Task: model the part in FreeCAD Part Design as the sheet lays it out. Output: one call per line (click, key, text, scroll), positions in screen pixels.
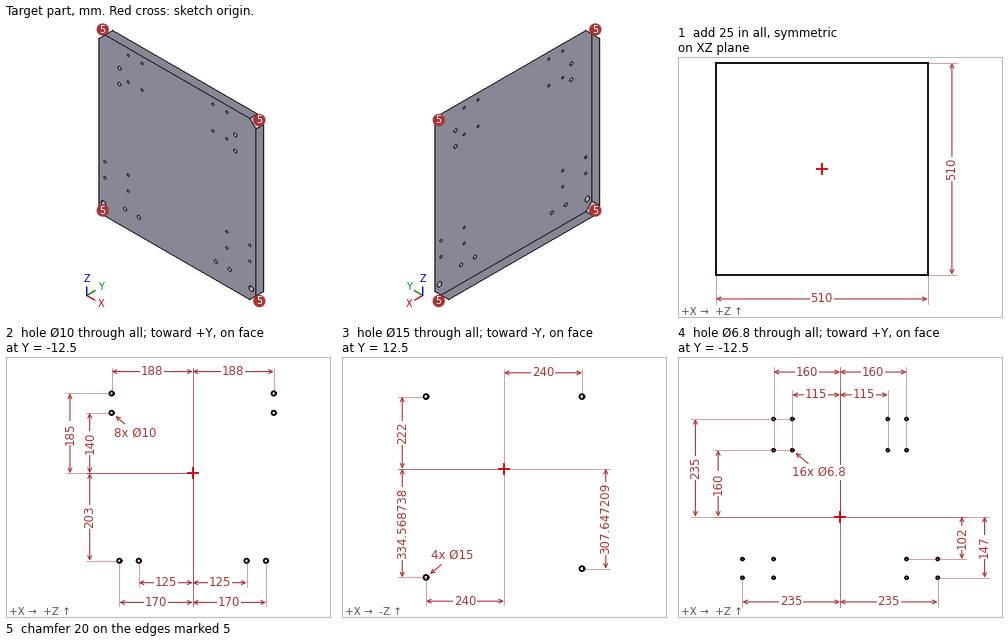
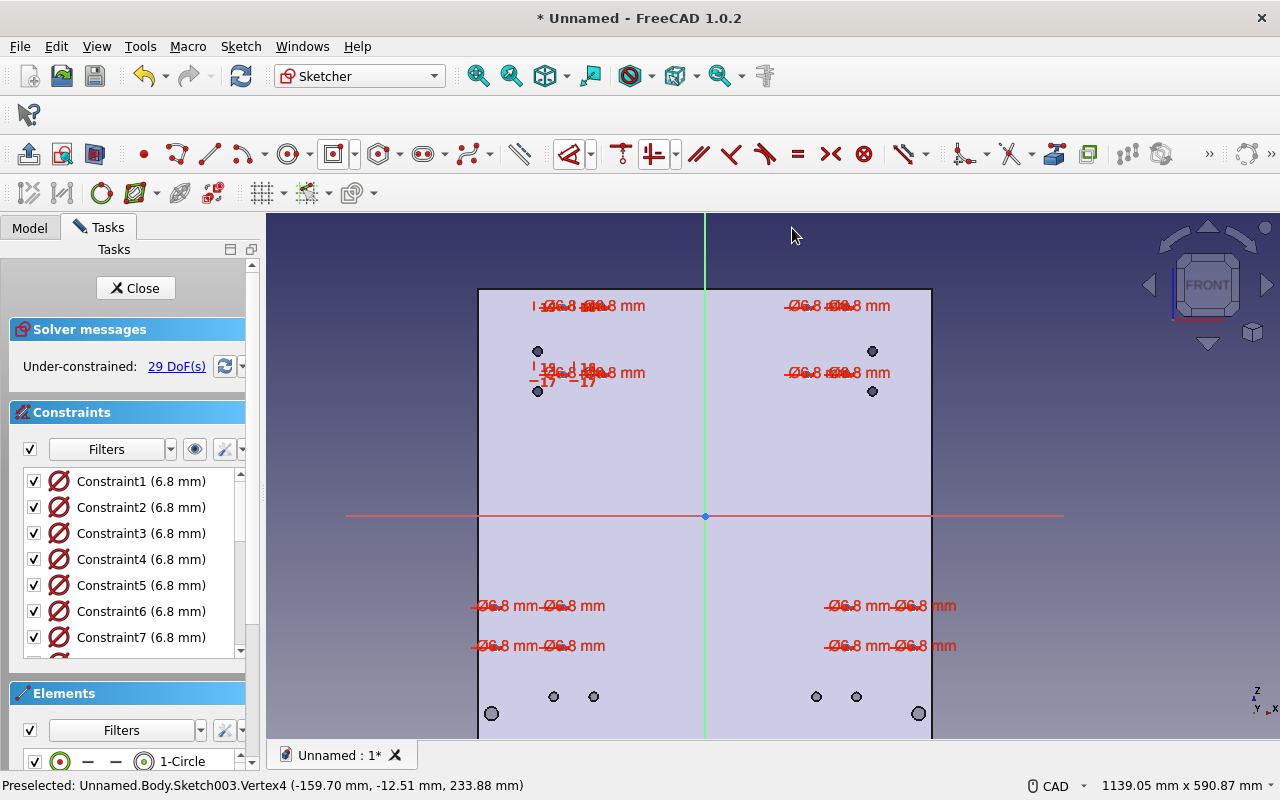
click(603, 308)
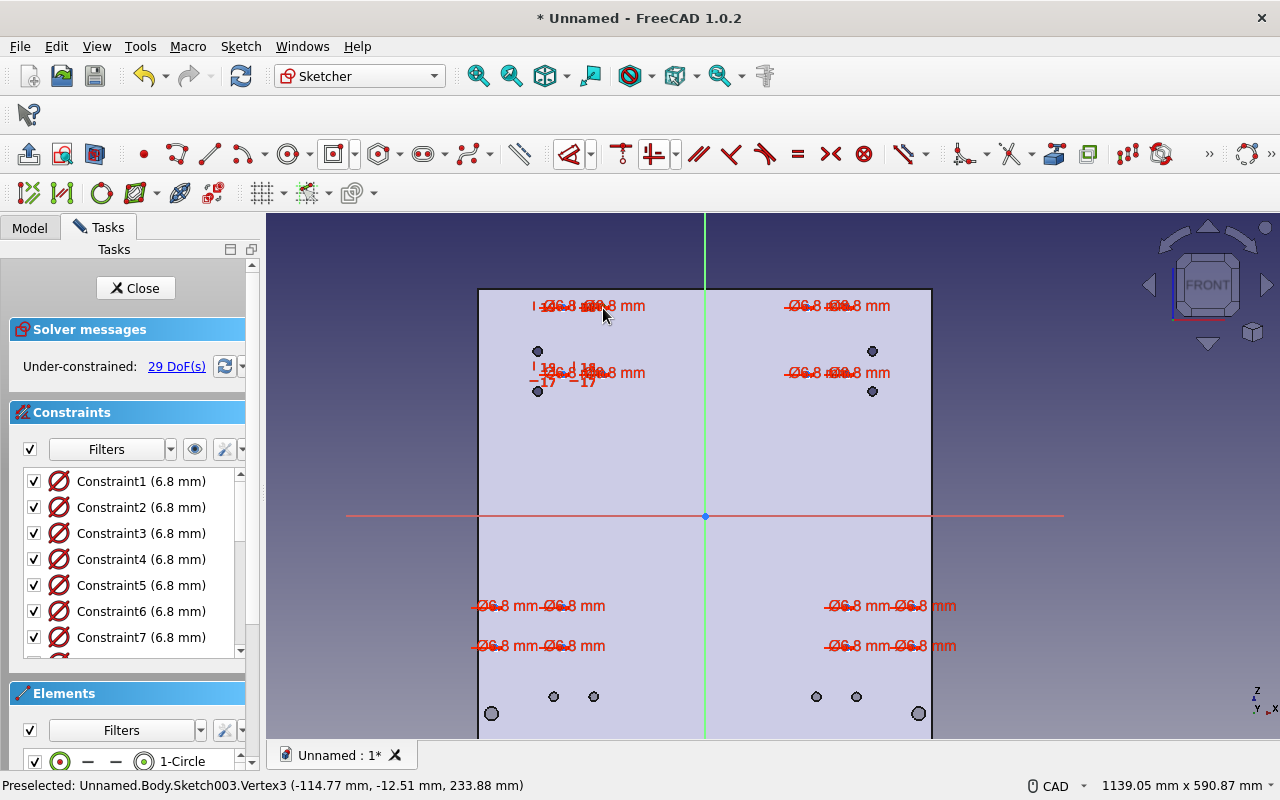
click(563, 308)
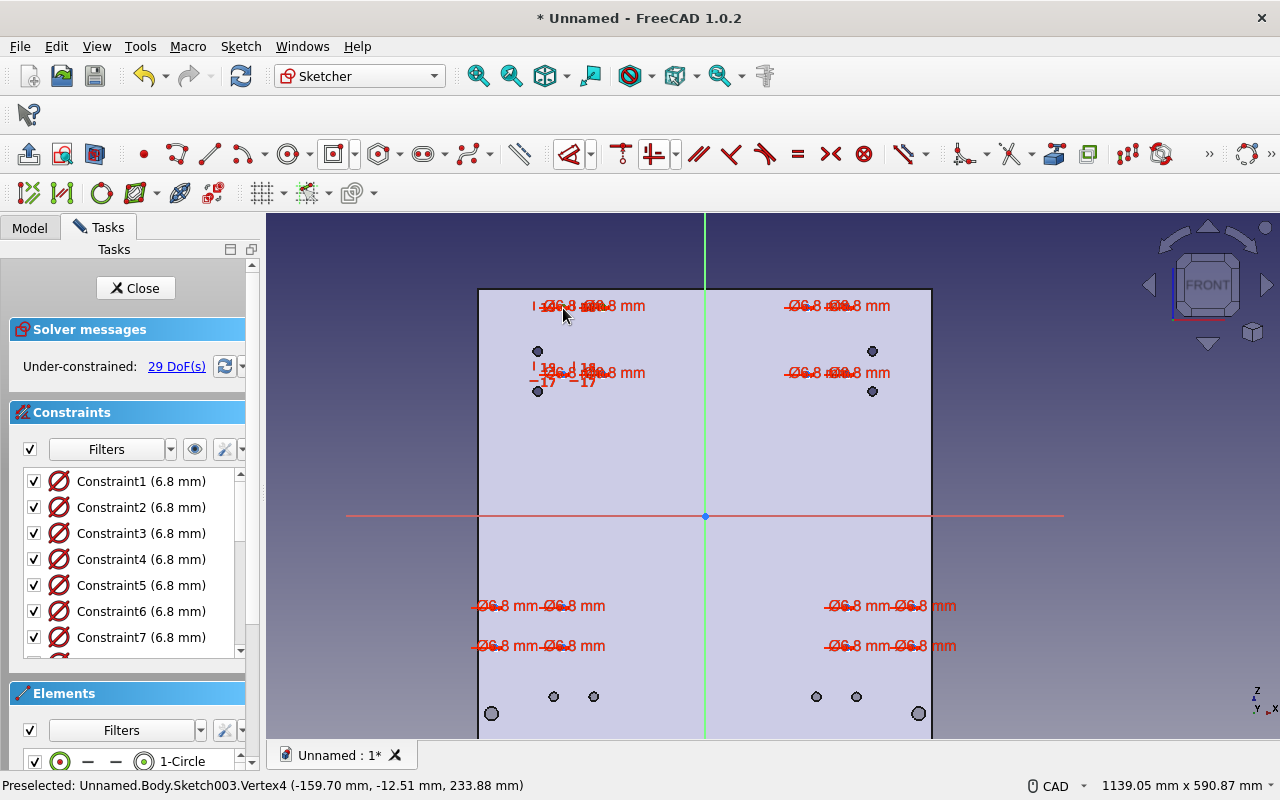
key(h)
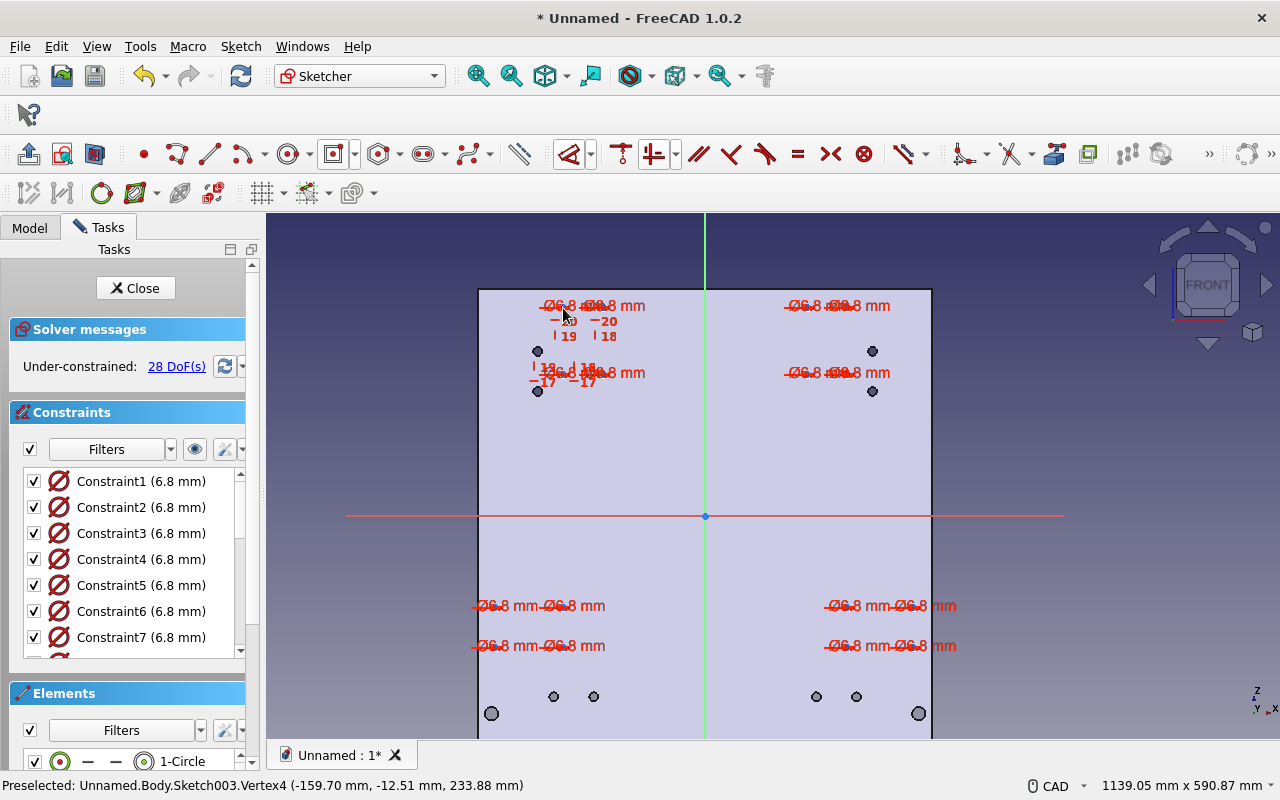
click(603, 375)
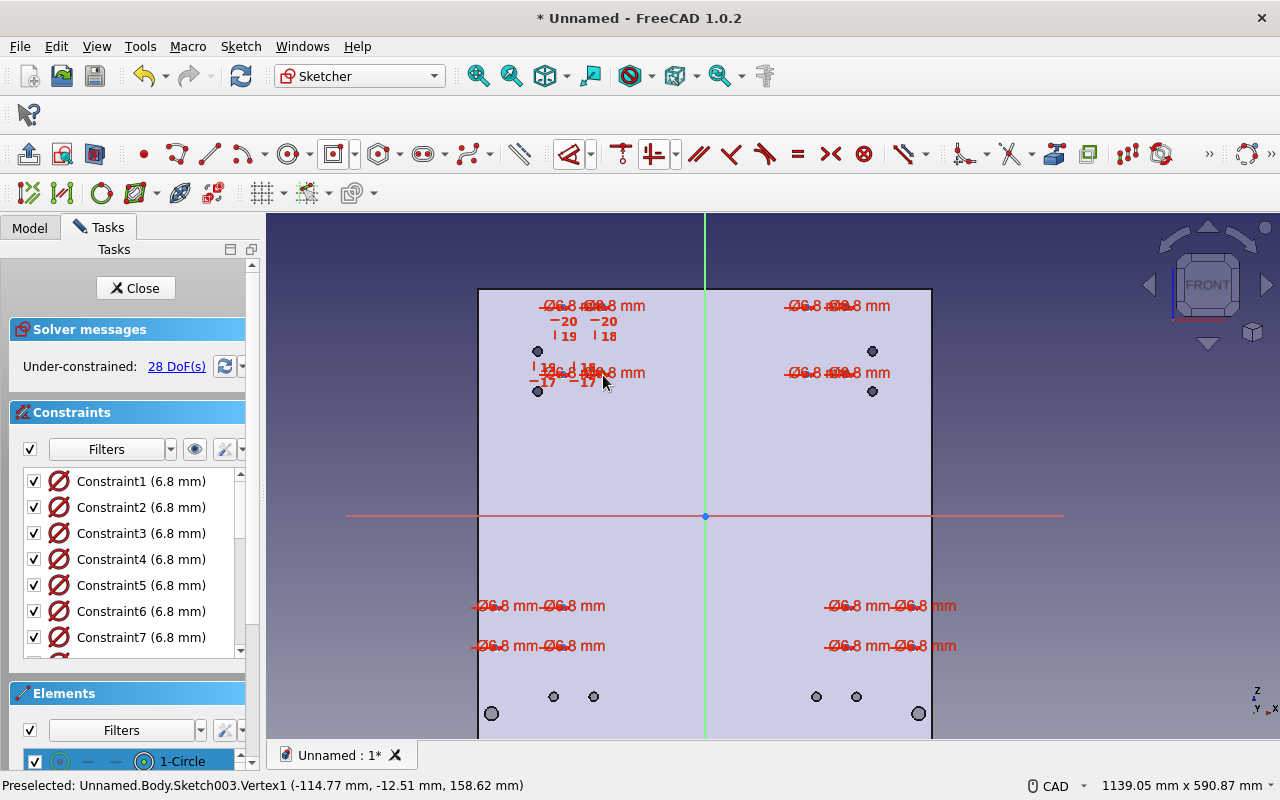
click(848, 375)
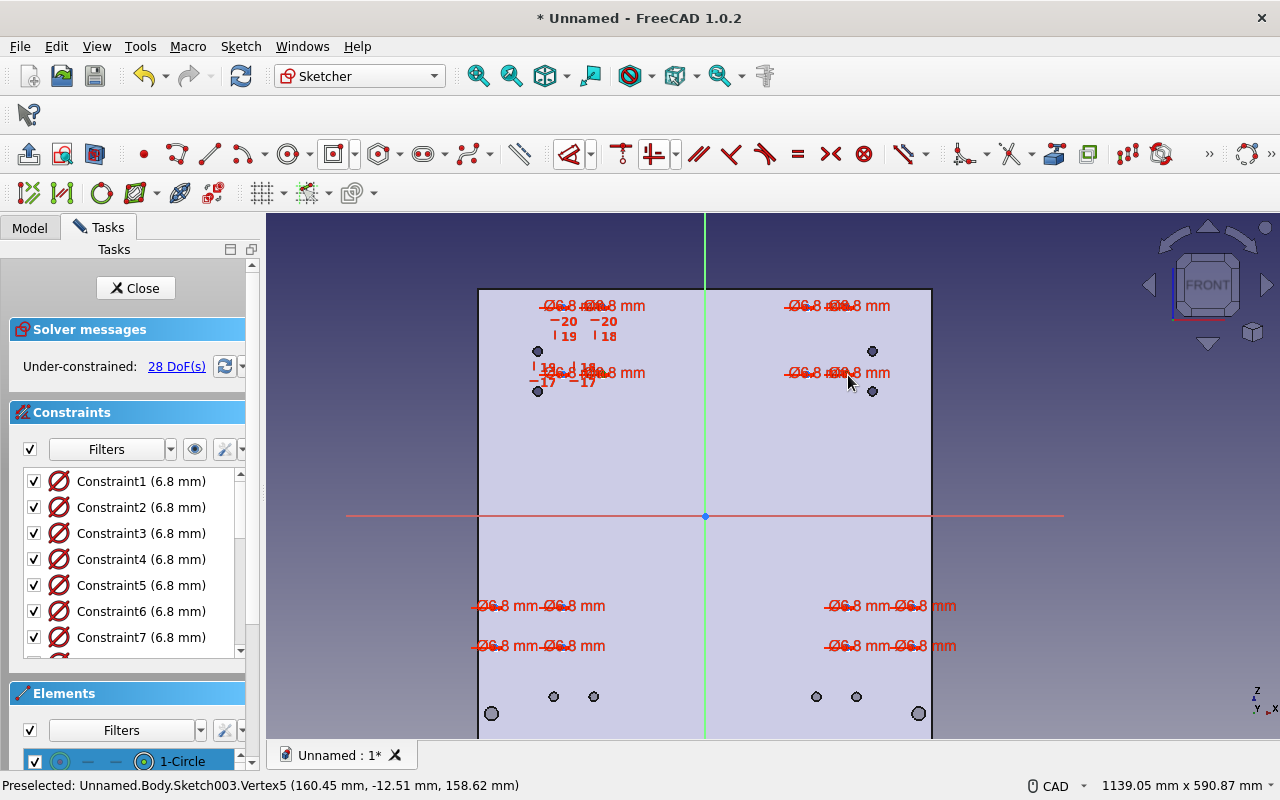
key(h)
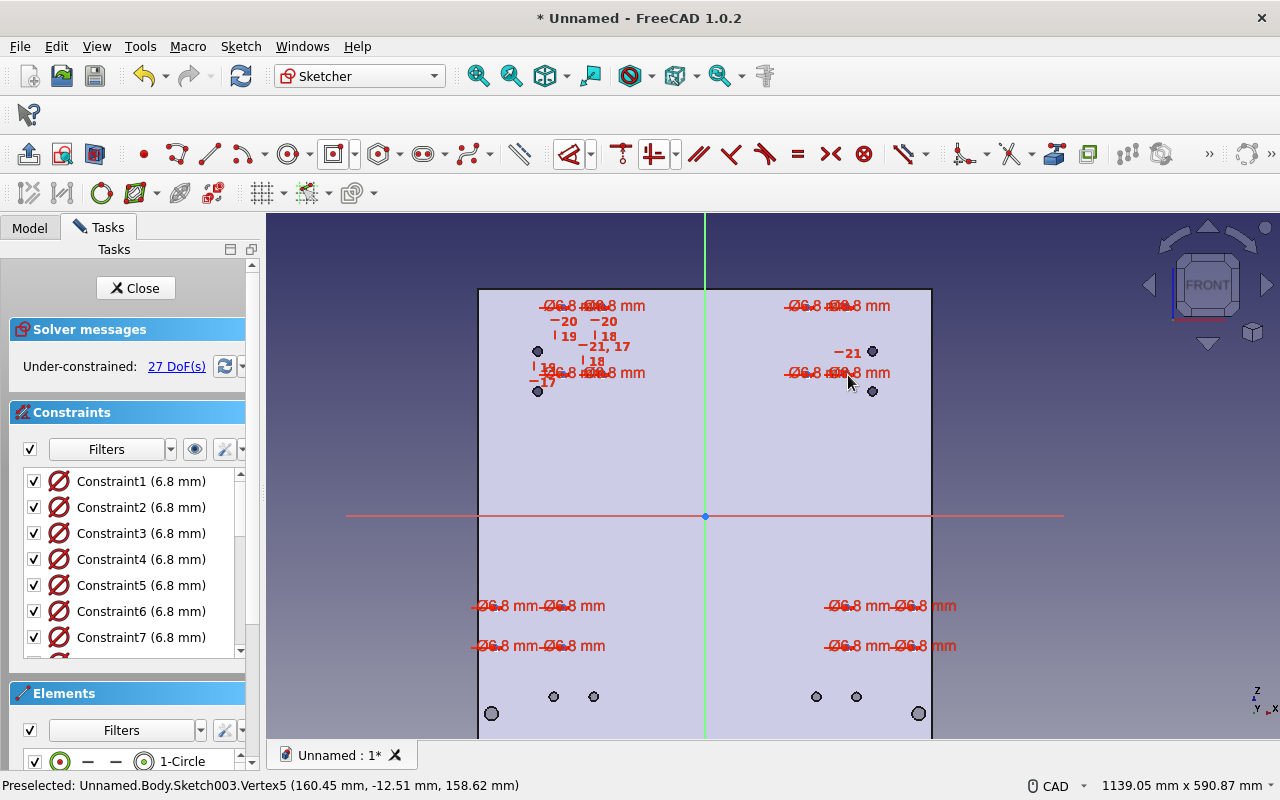
click(848, 375)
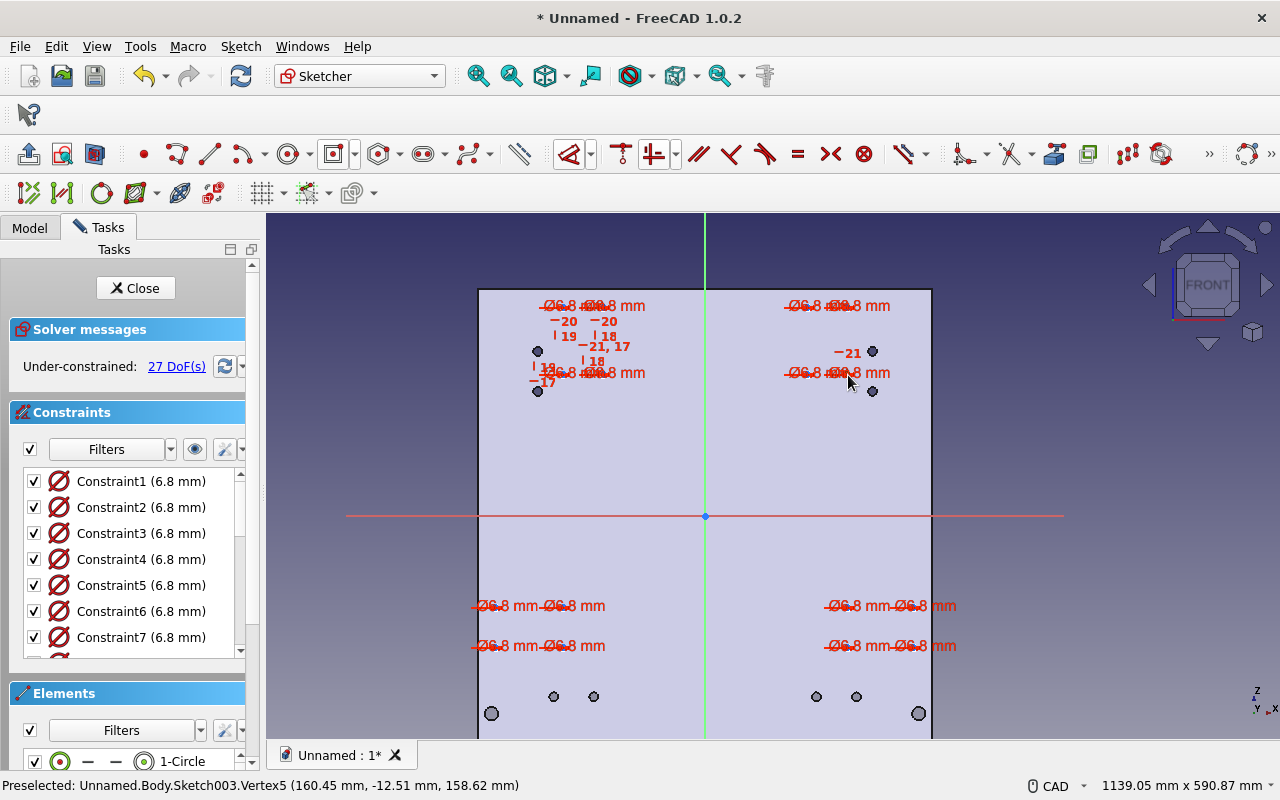
click(808, 375)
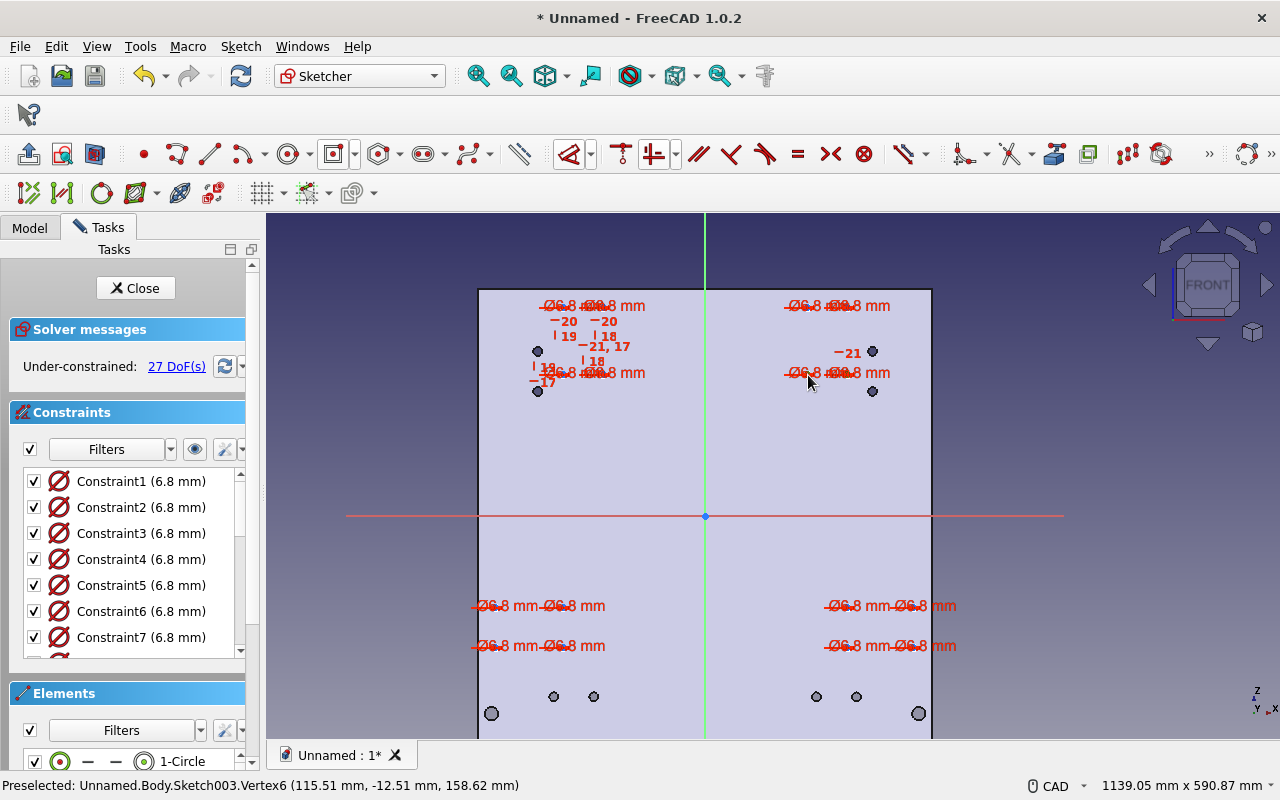
key(h)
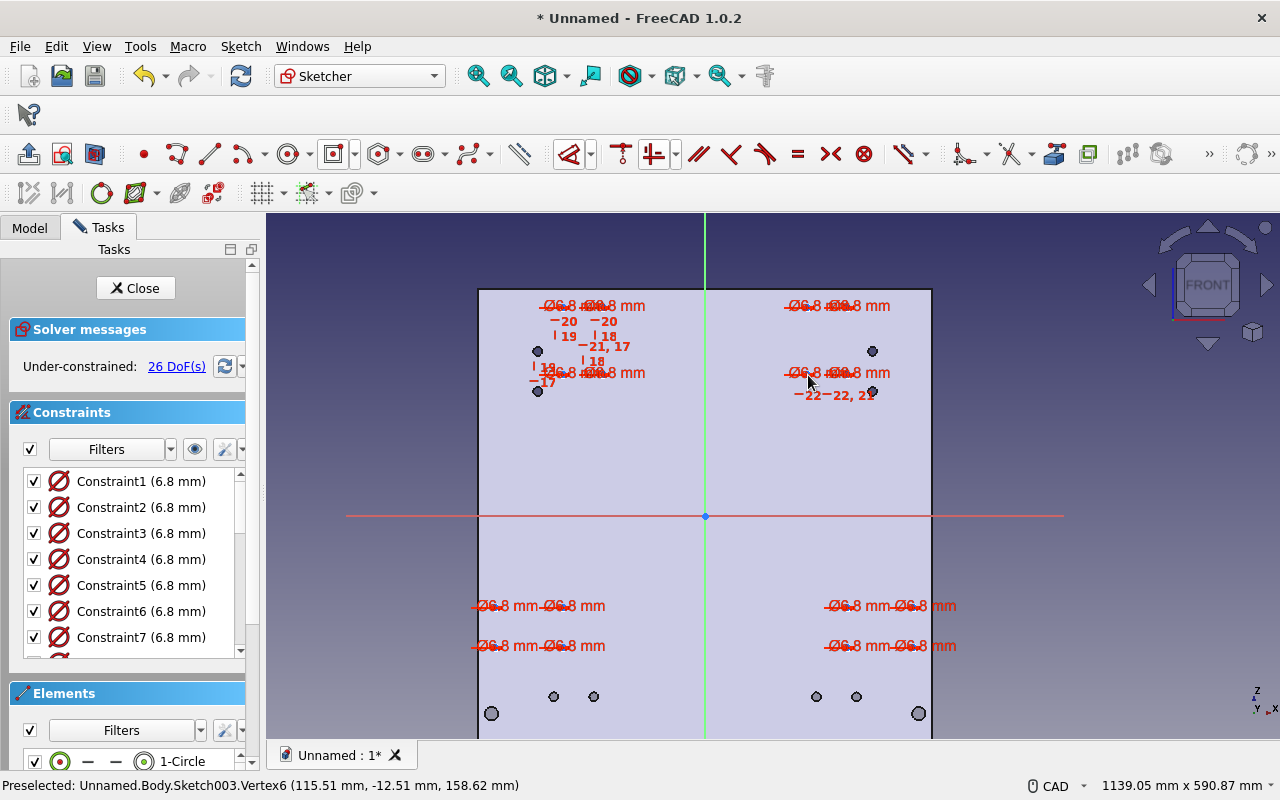
click(808, 375)